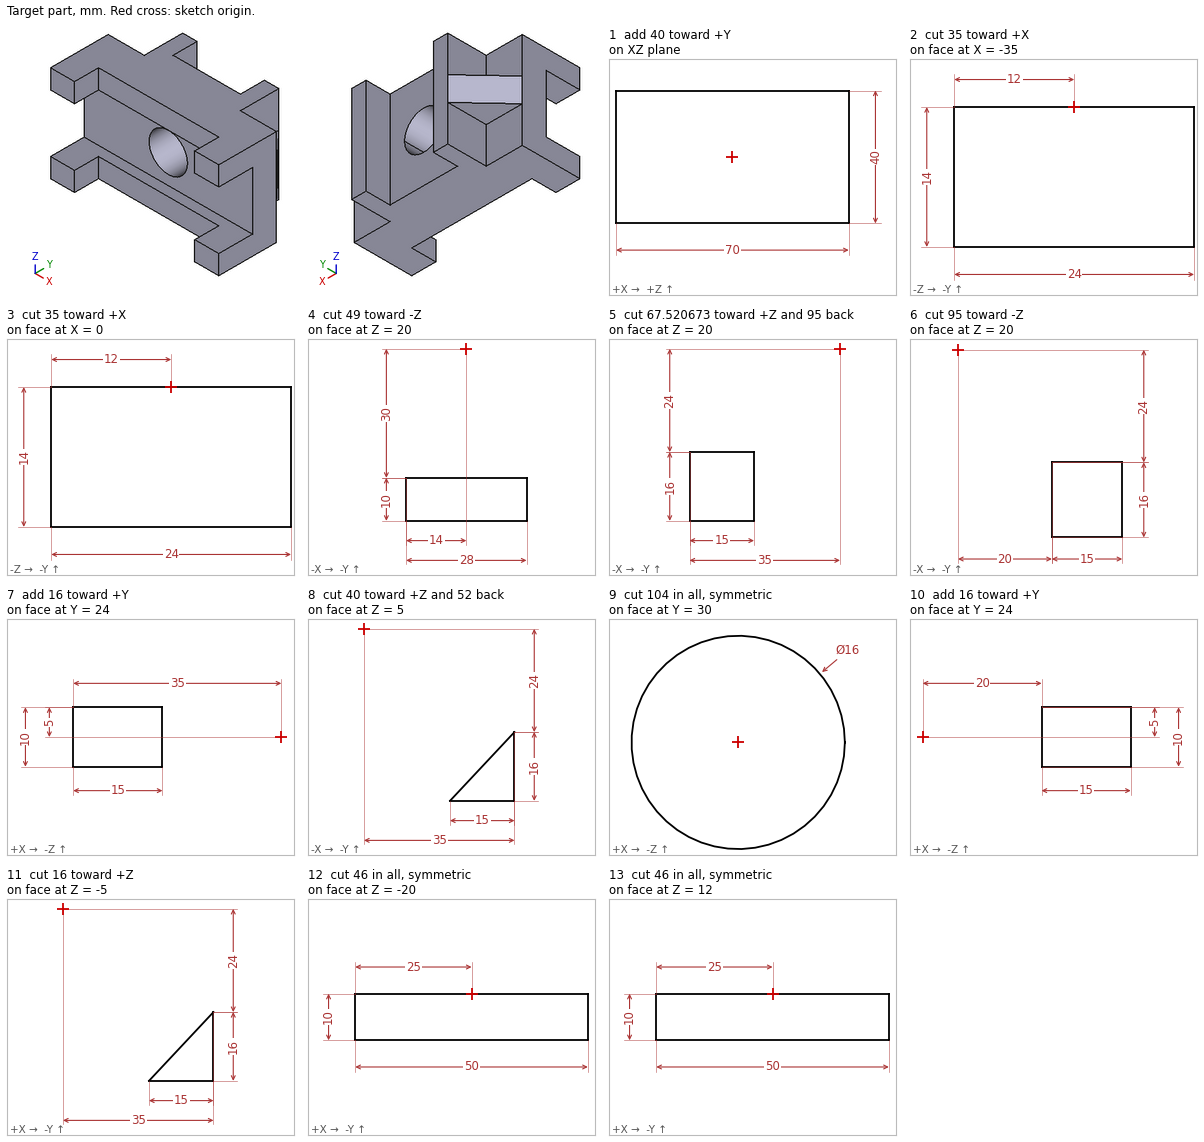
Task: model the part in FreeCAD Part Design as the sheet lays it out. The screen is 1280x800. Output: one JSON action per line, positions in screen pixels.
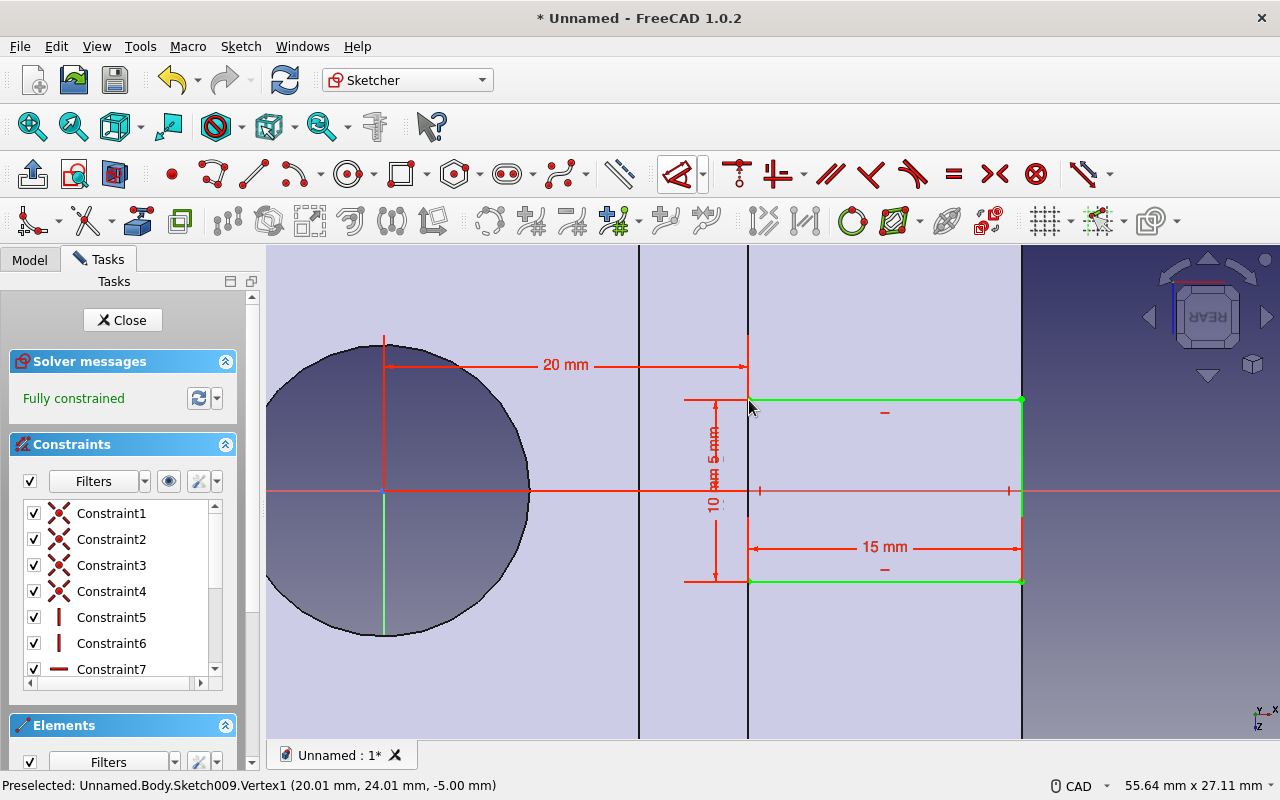
{"action": "left_click", "coordinate": [123, 320]}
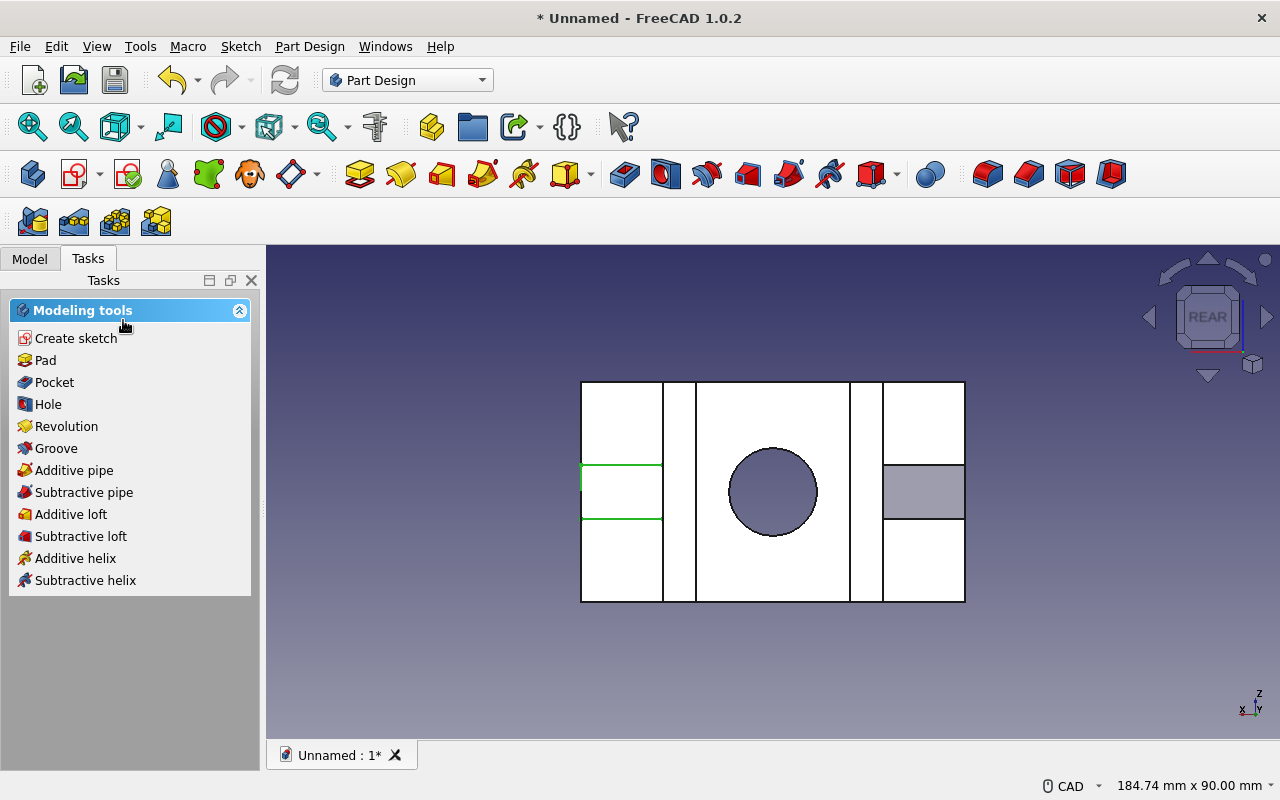
{"action": "left_click", "coordinate": [360, 174]}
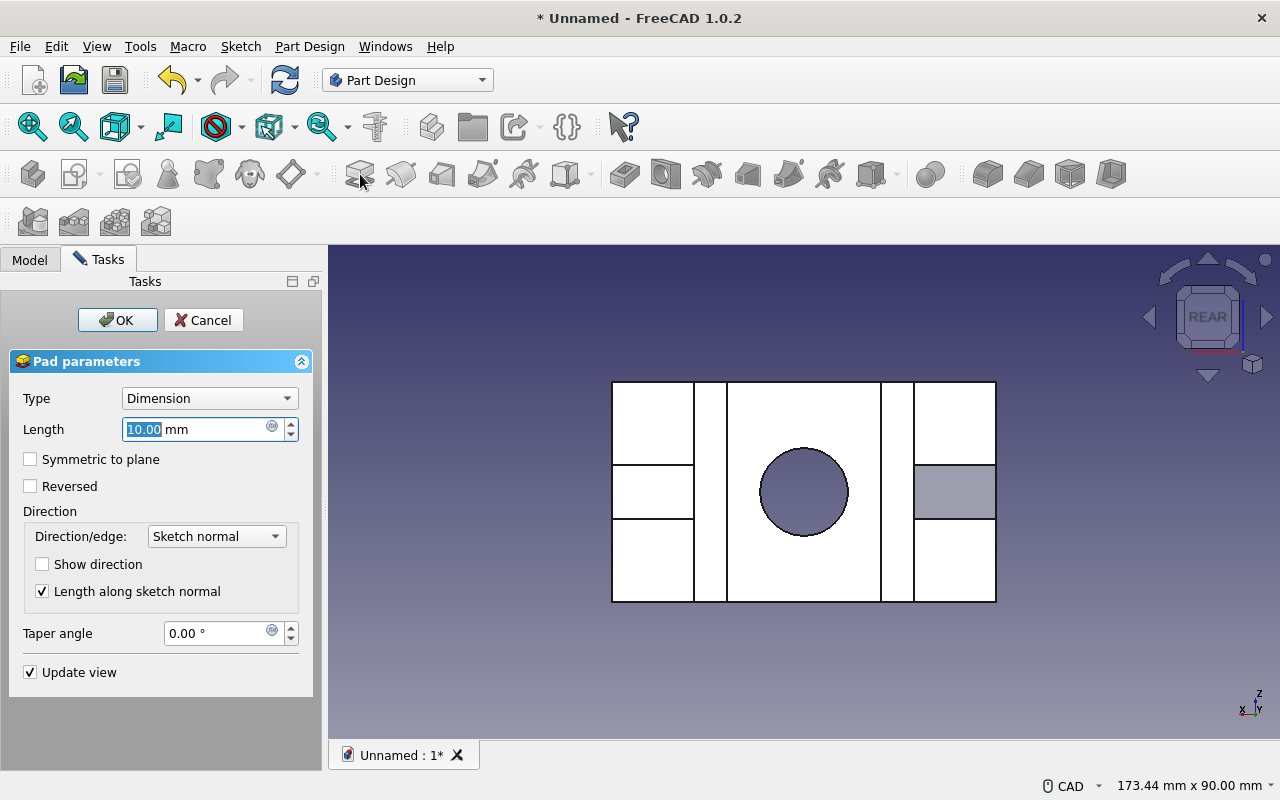
{"action": "type", "text": "16"}
{"action": "key", "text": "Tab"}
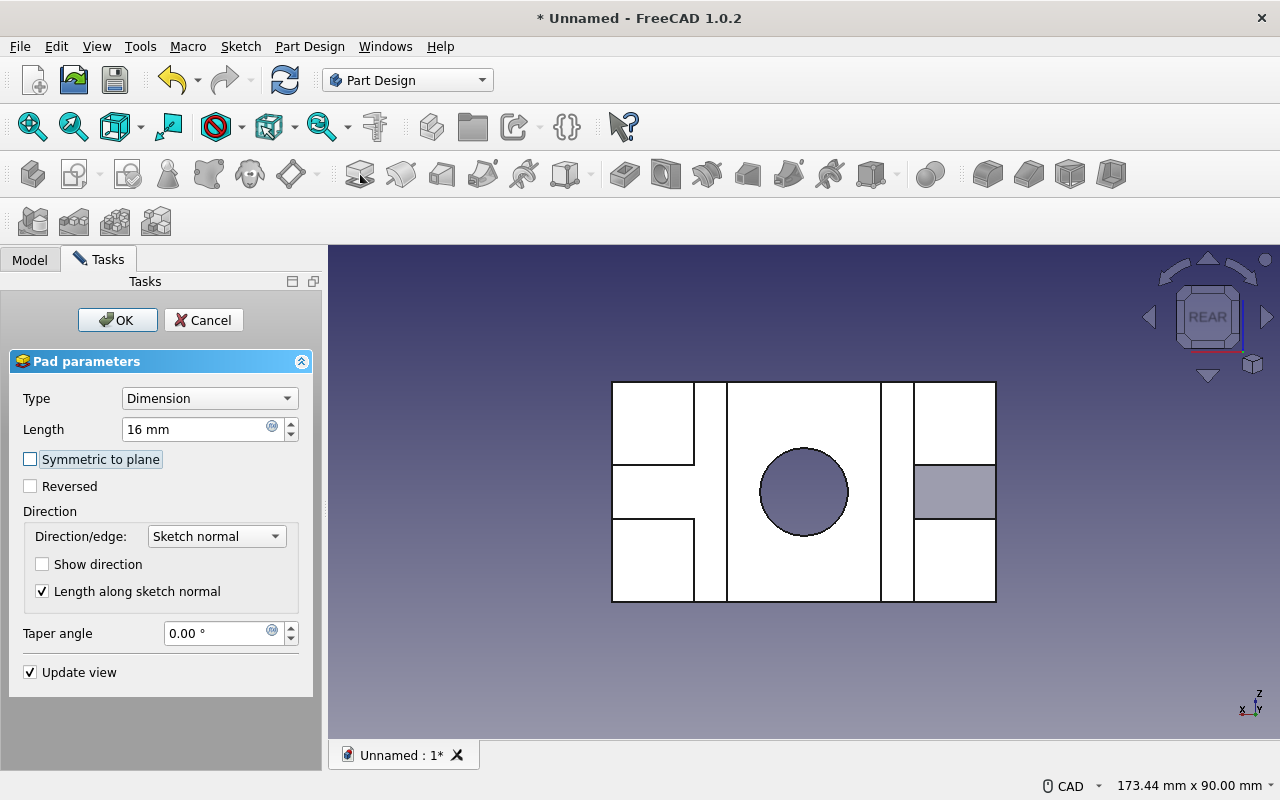
{"action": "left_click", "coordinate": [118, 320]}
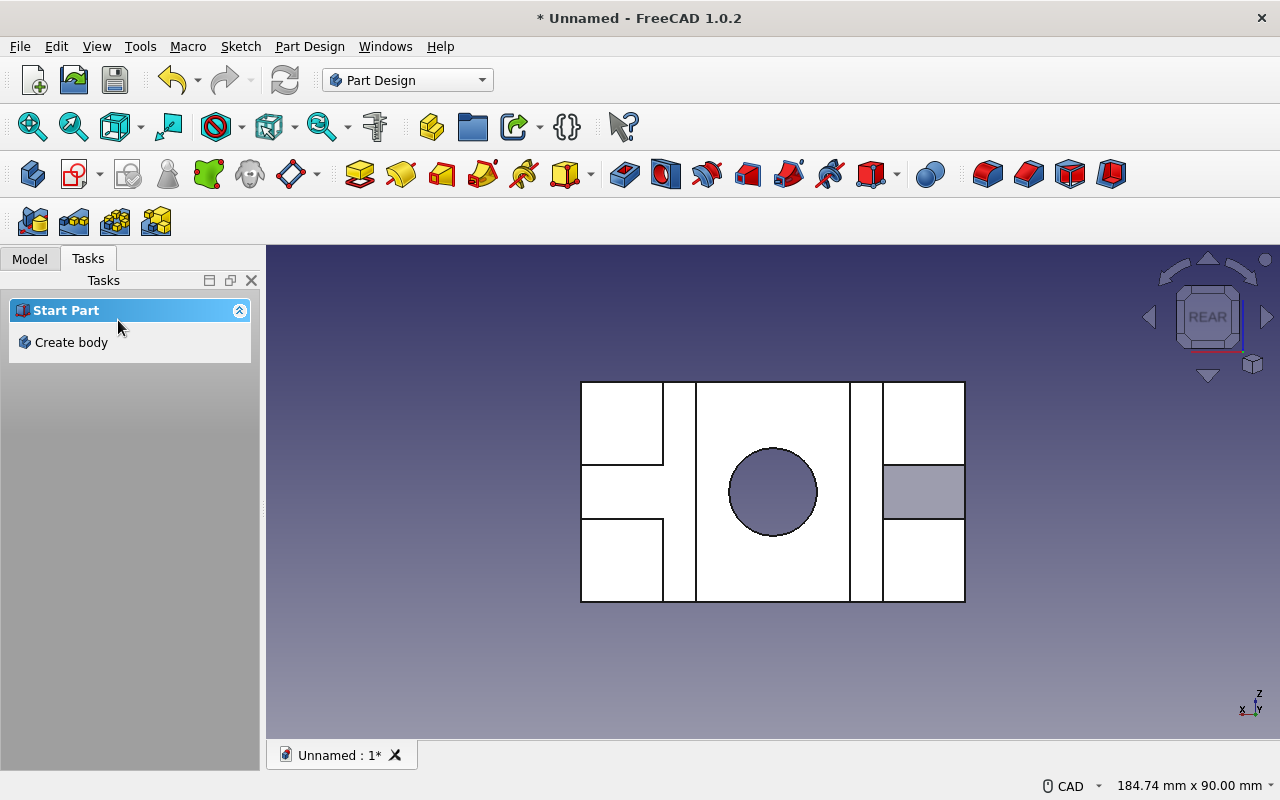
{"action": "key", "text": "v f"}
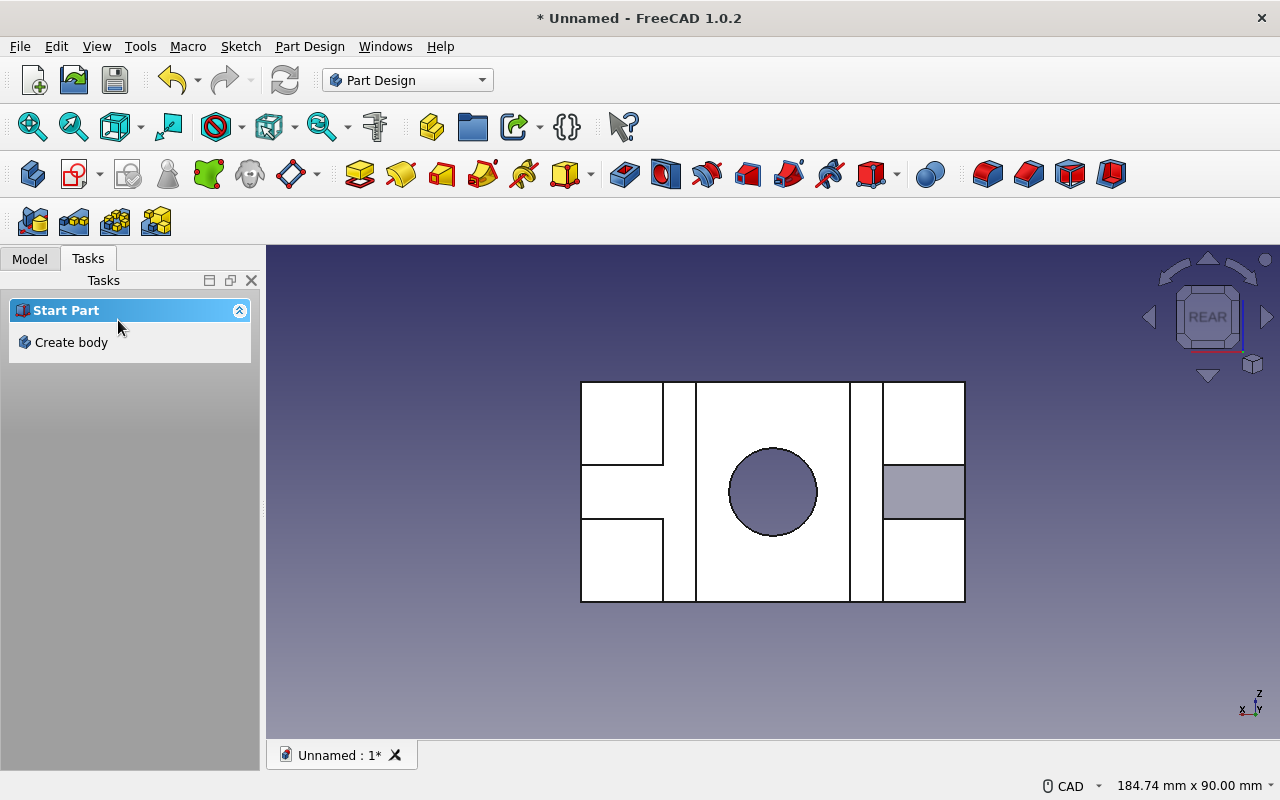
{"action": "key", "text": "5"}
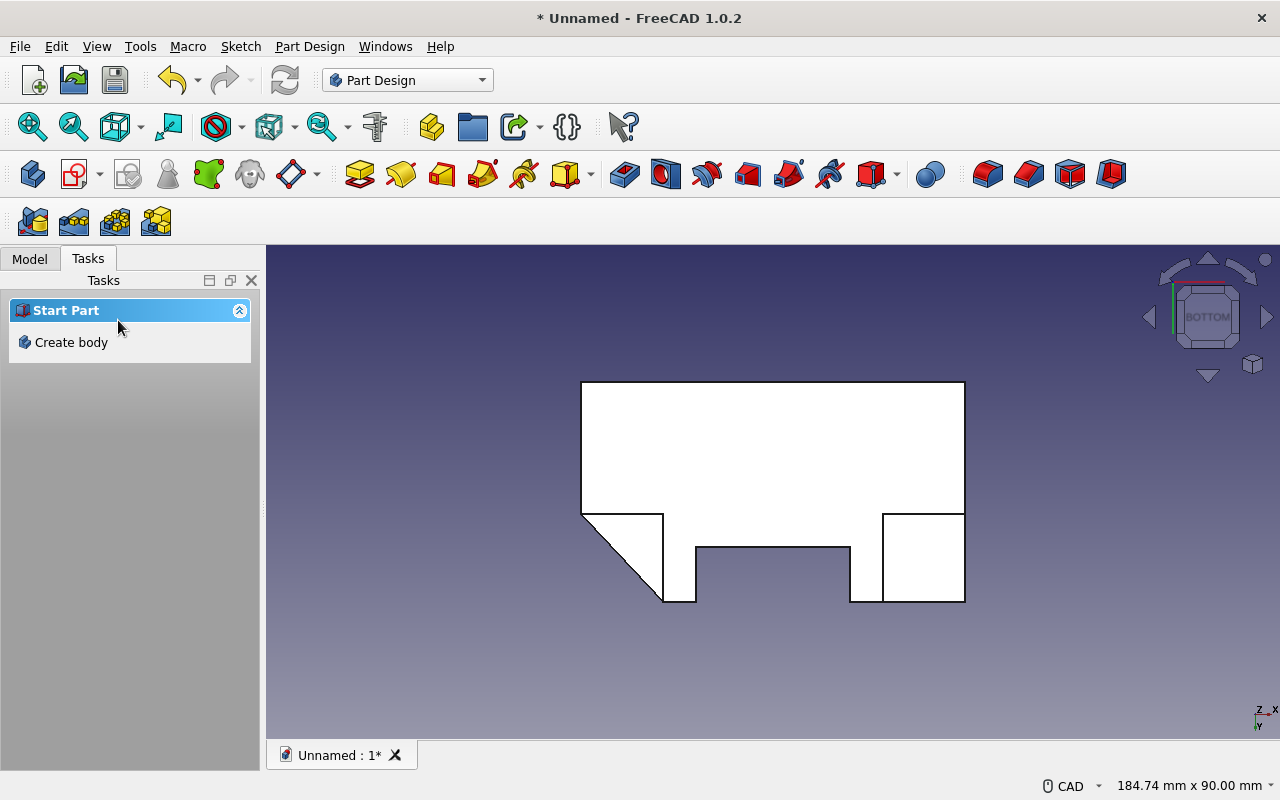
{"action": "key", "text": "v f"}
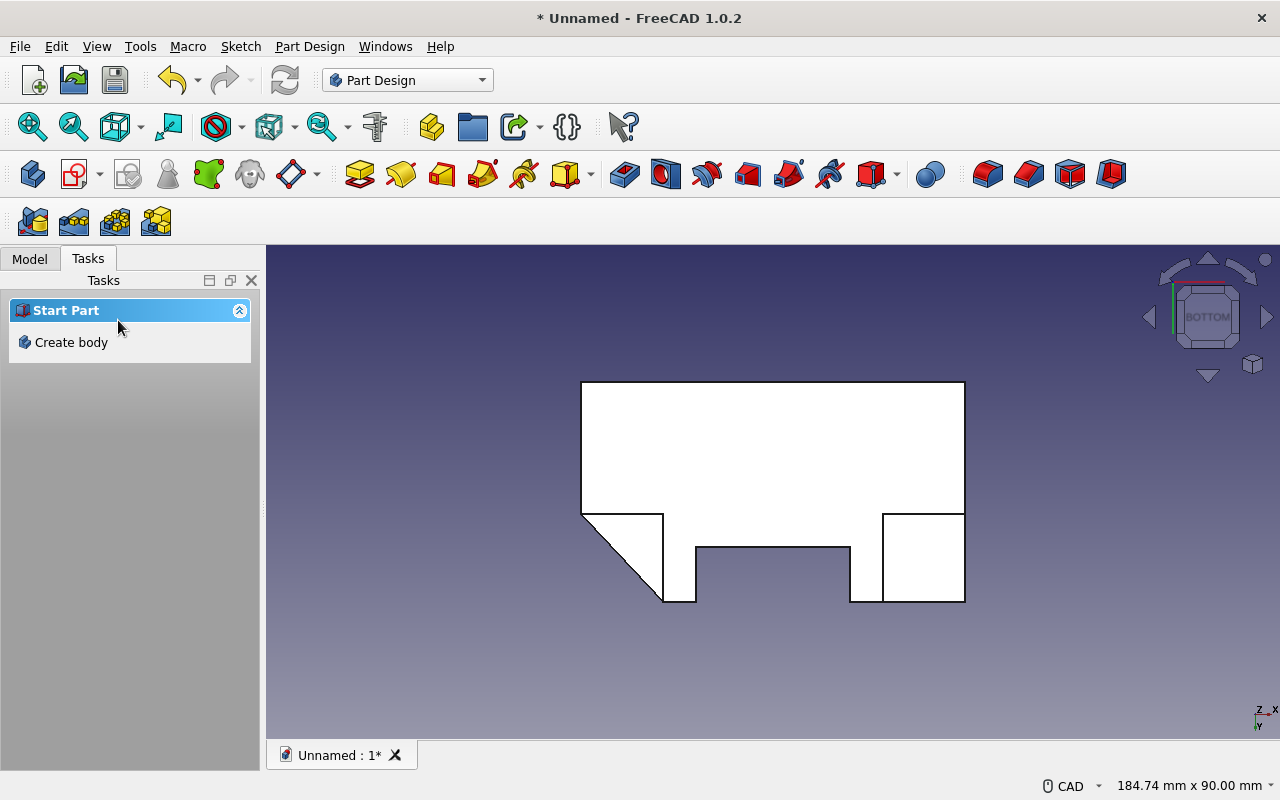
{"action": "left_click", "coordinate": [924, 557]}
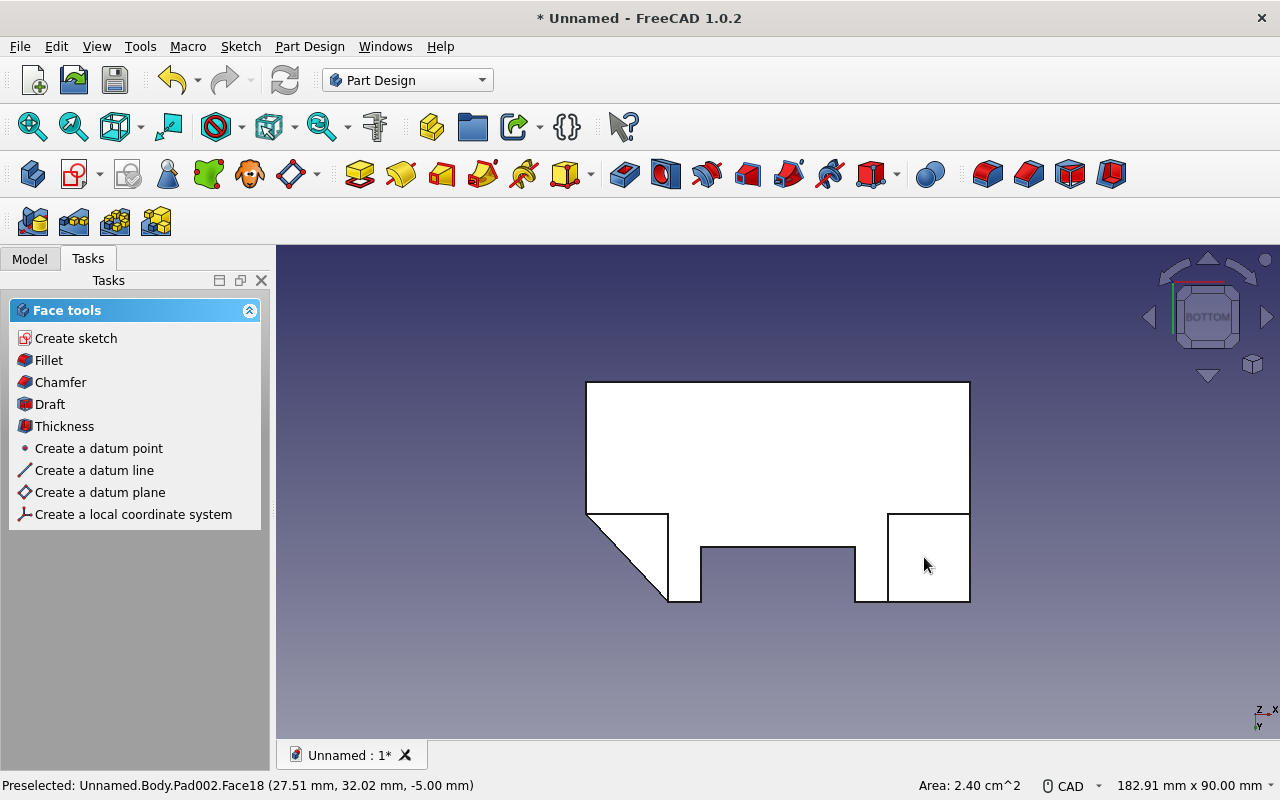
{"action": "left_click", "coordinate": [74, 174]}